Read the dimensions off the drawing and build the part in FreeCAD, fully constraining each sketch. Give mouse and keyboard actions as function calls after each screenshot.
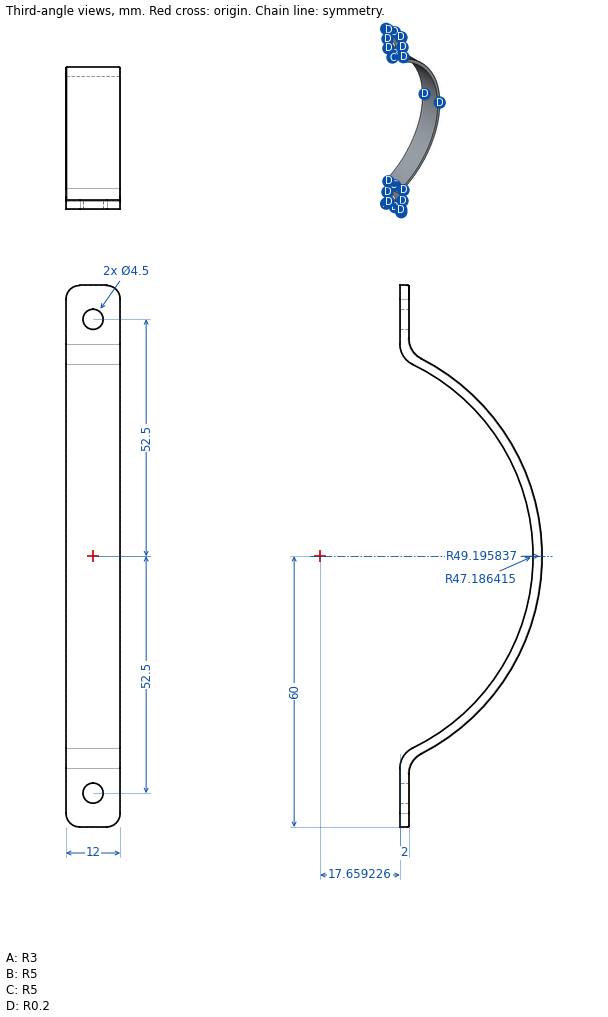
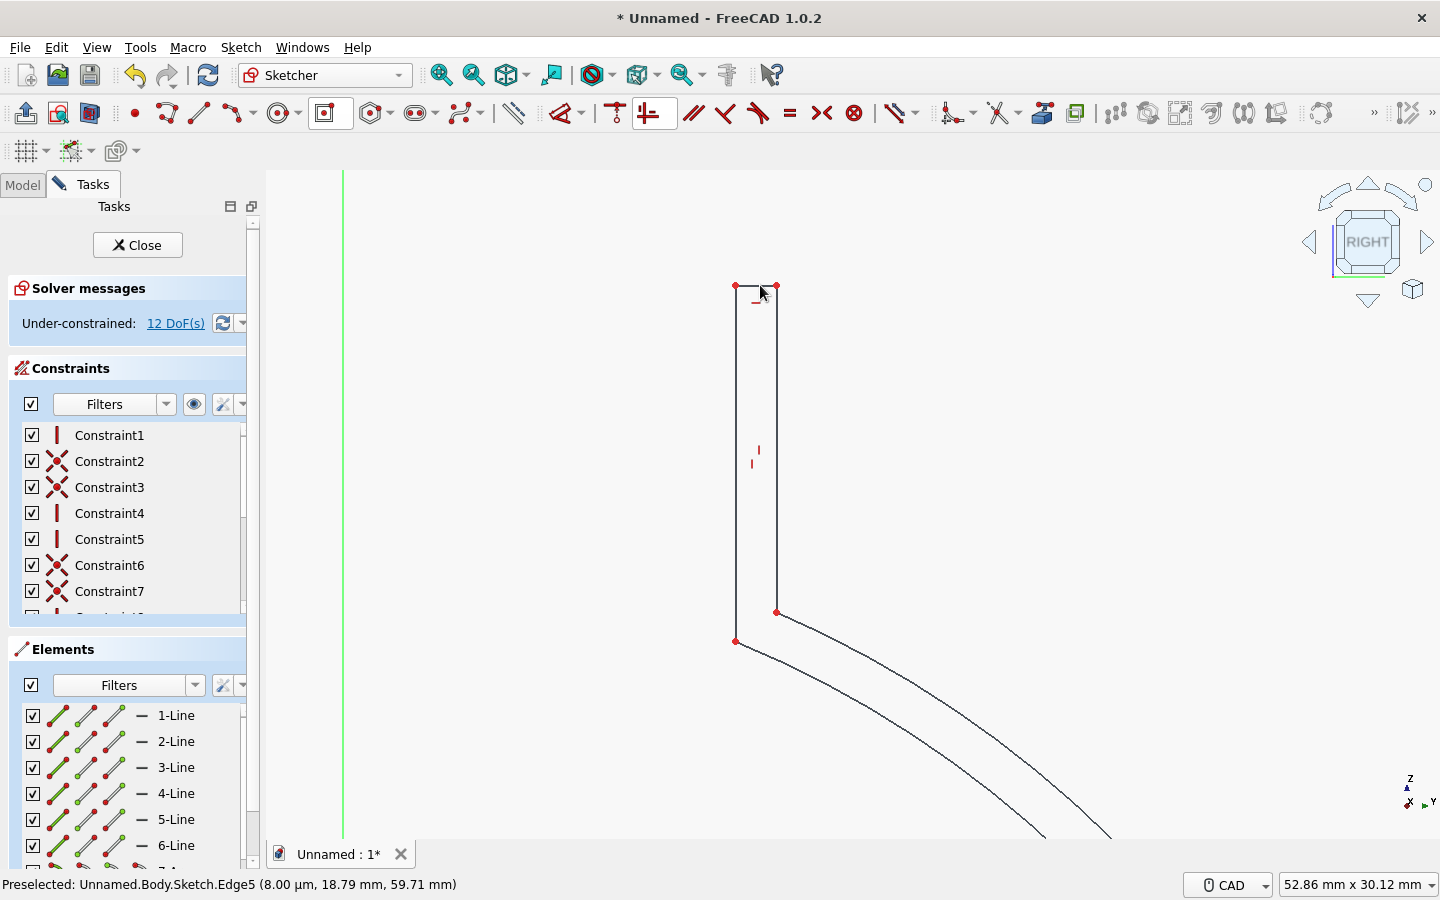
scroll(764, 285, down, 9)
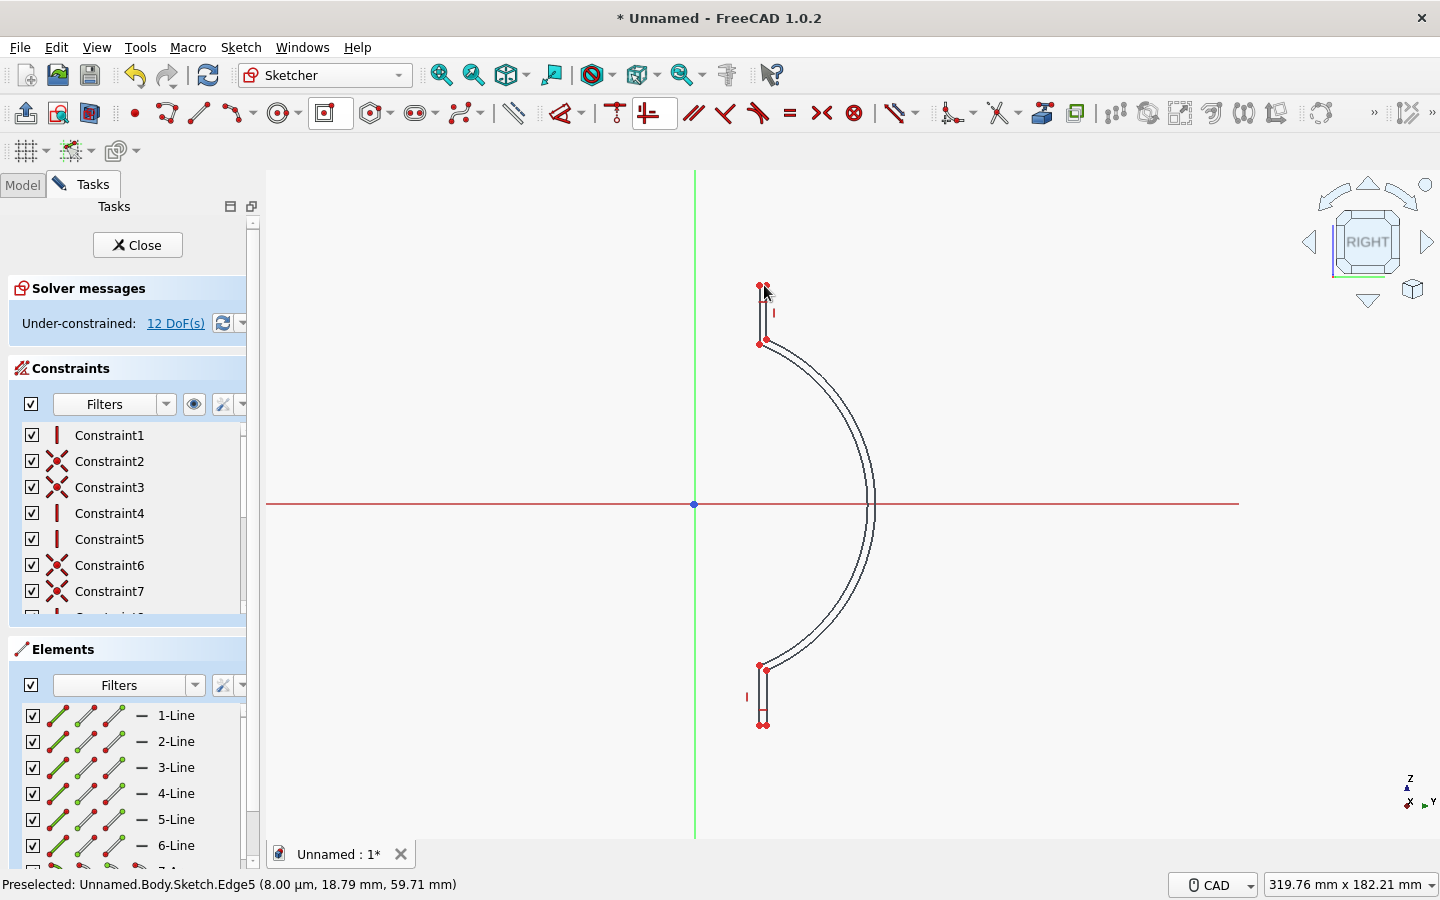
scroll(856, 586, up, 3)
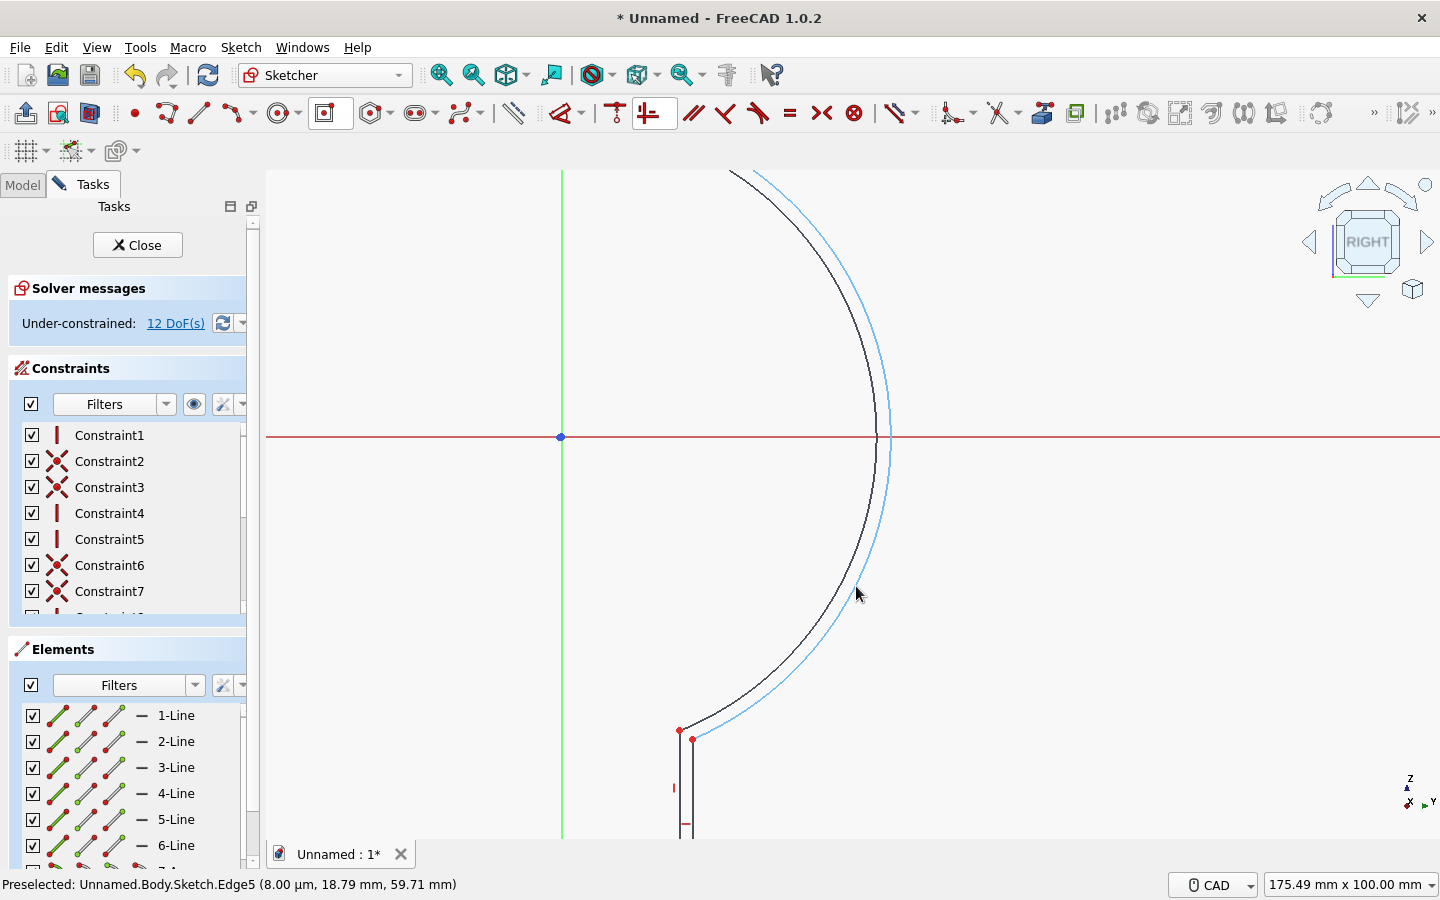
click(856, 585)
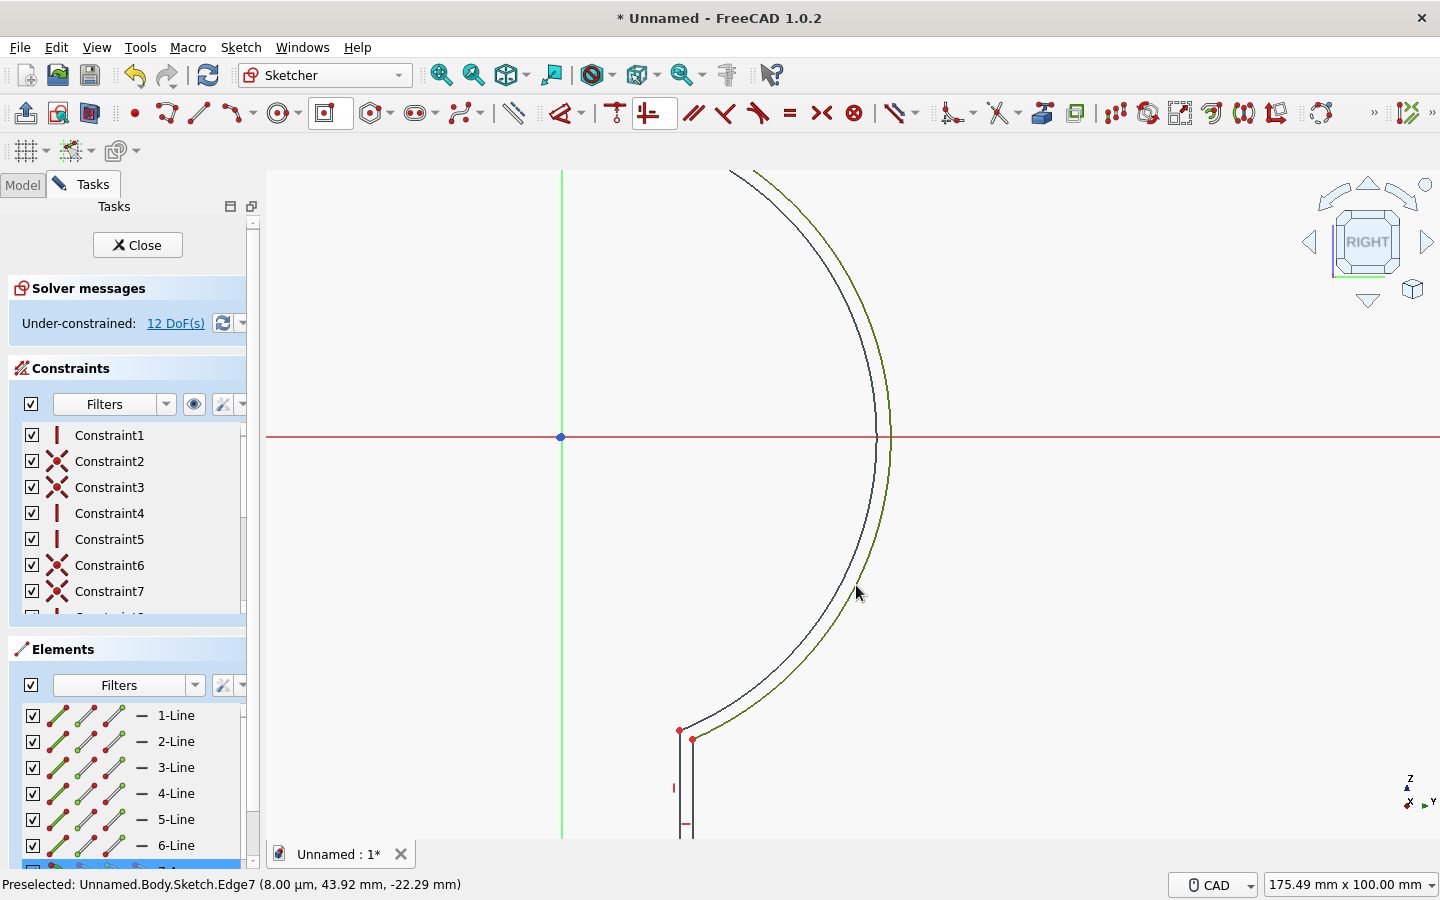
click(842, 582)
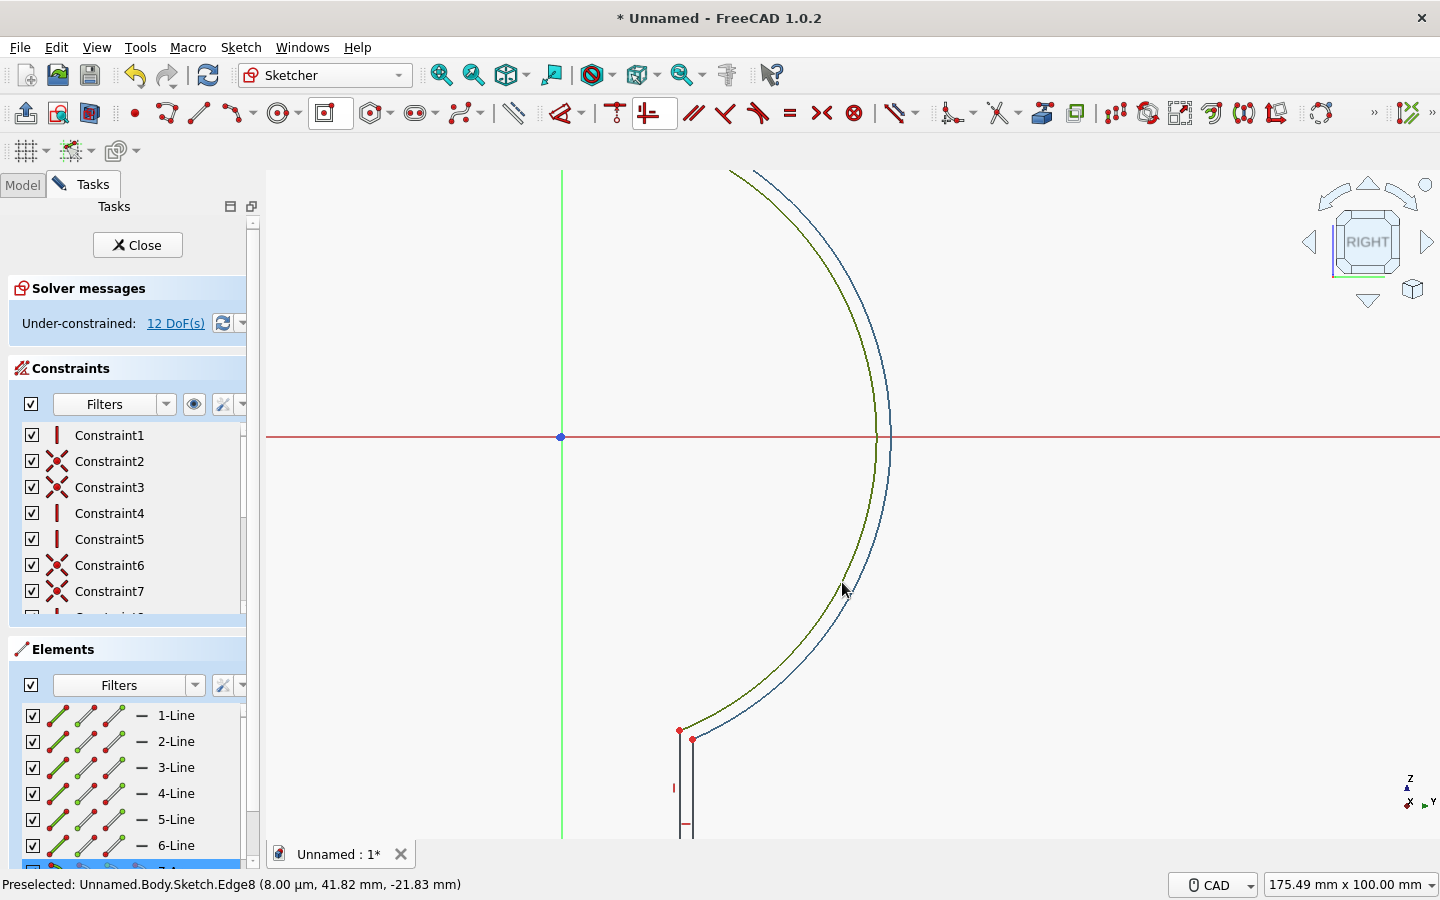
click(616, 114)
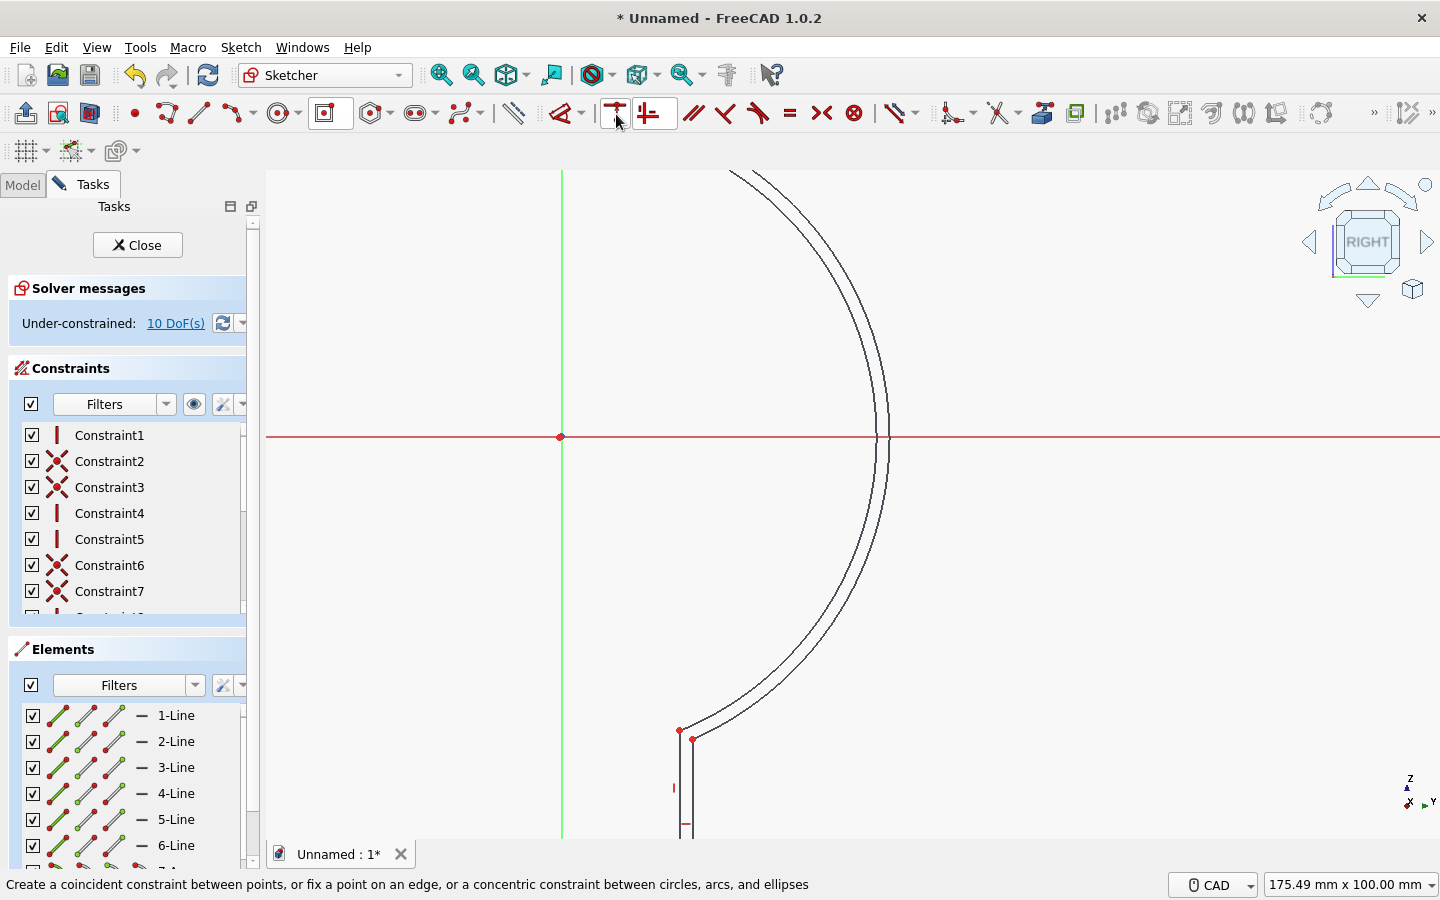
drag(550, 427, 572, 448)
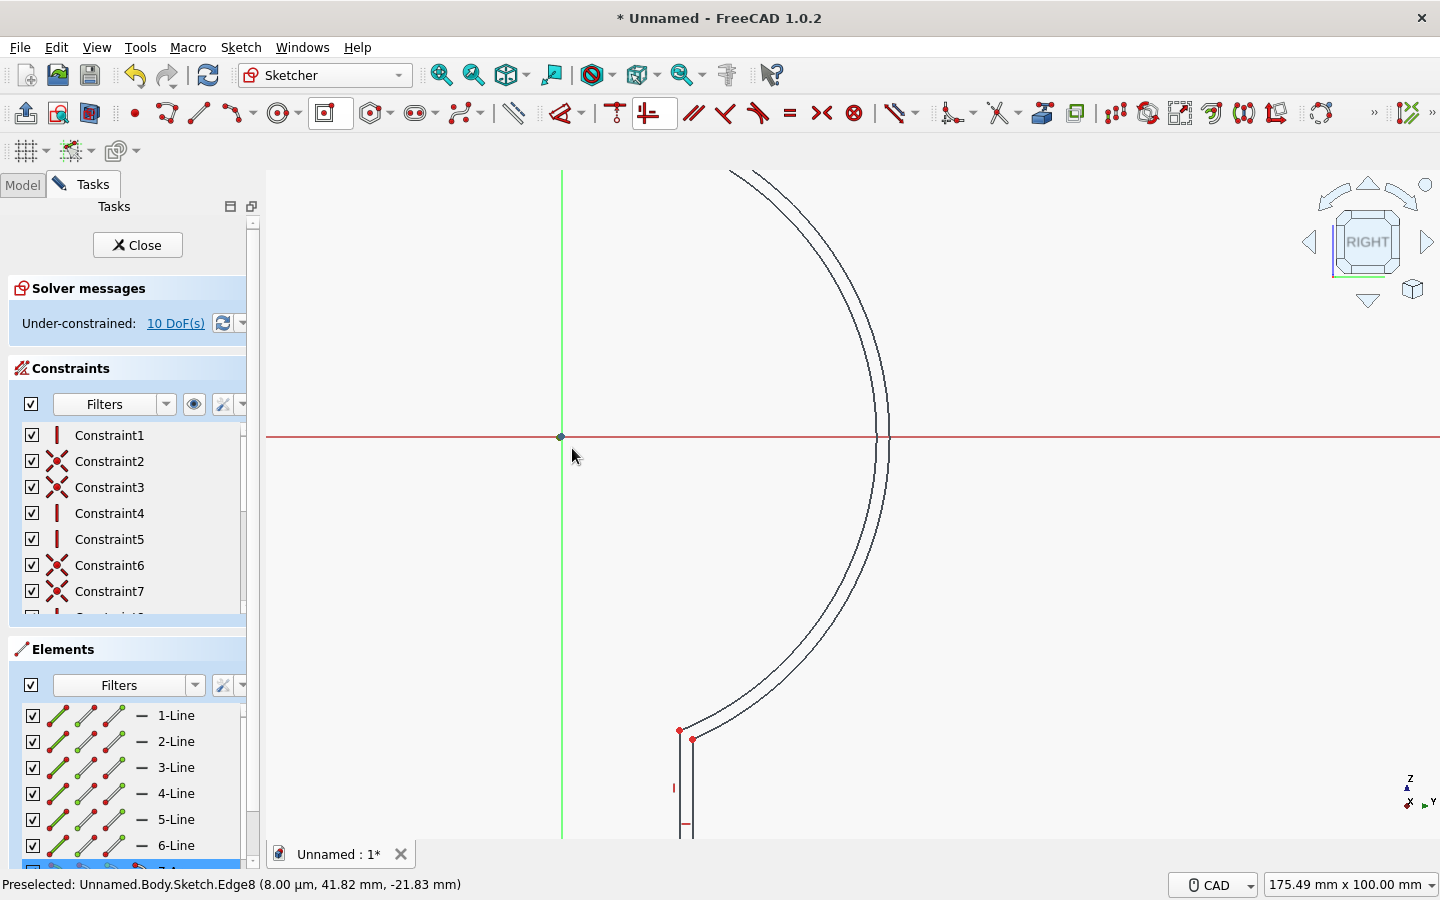
click(616, 114)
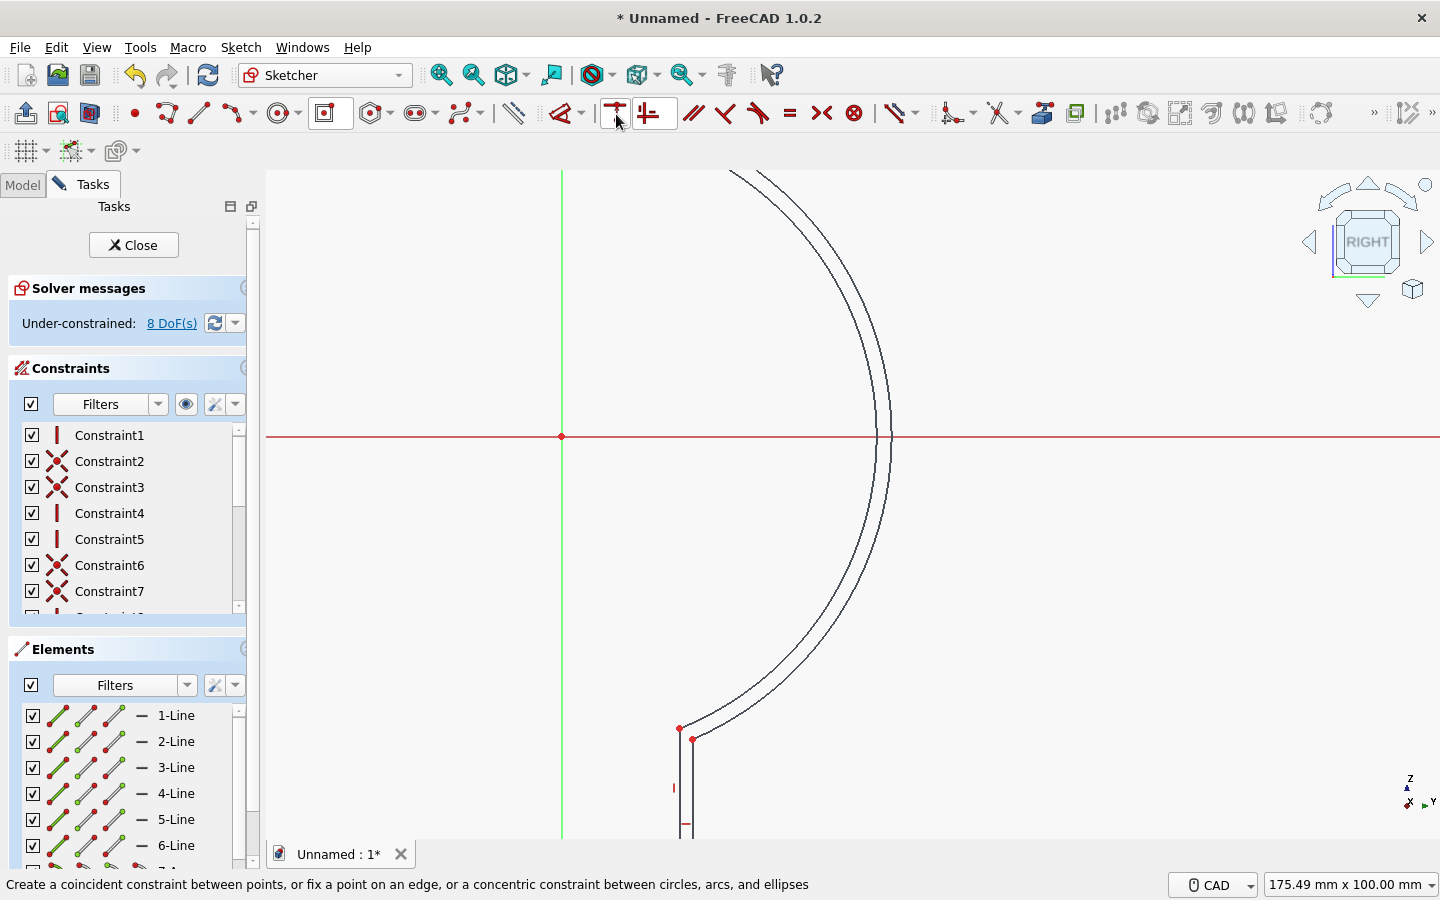
scroll(855, 587, down, 3)